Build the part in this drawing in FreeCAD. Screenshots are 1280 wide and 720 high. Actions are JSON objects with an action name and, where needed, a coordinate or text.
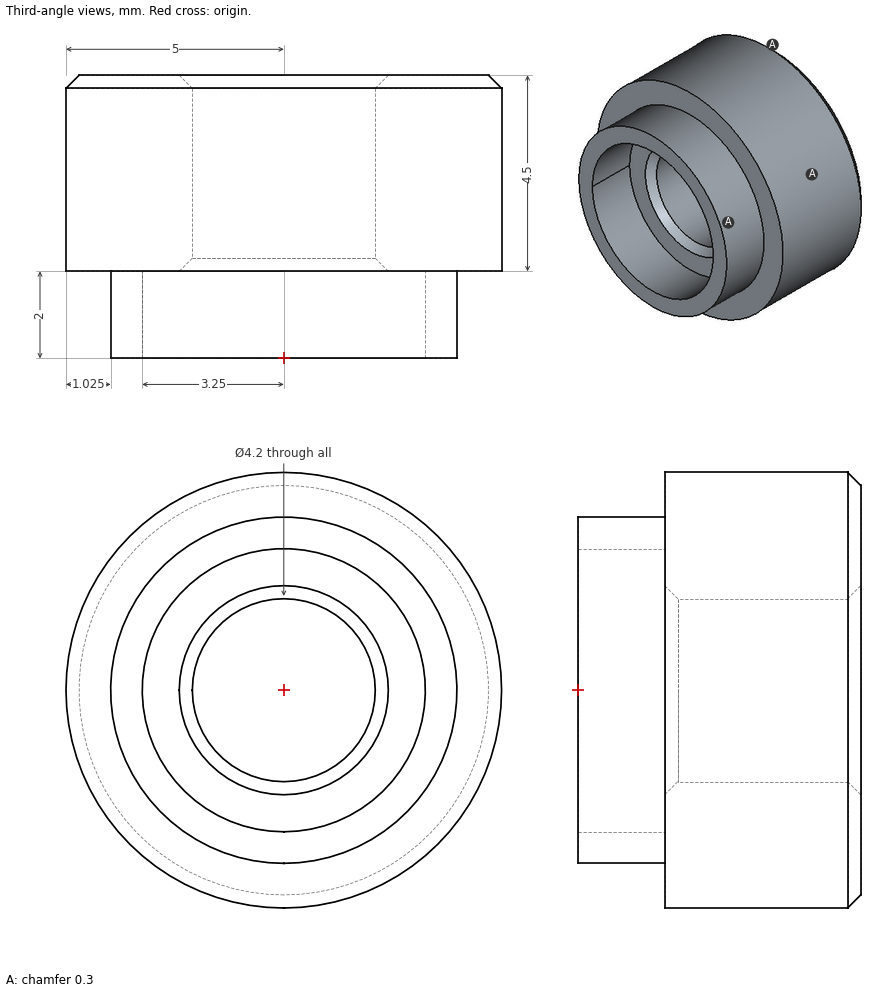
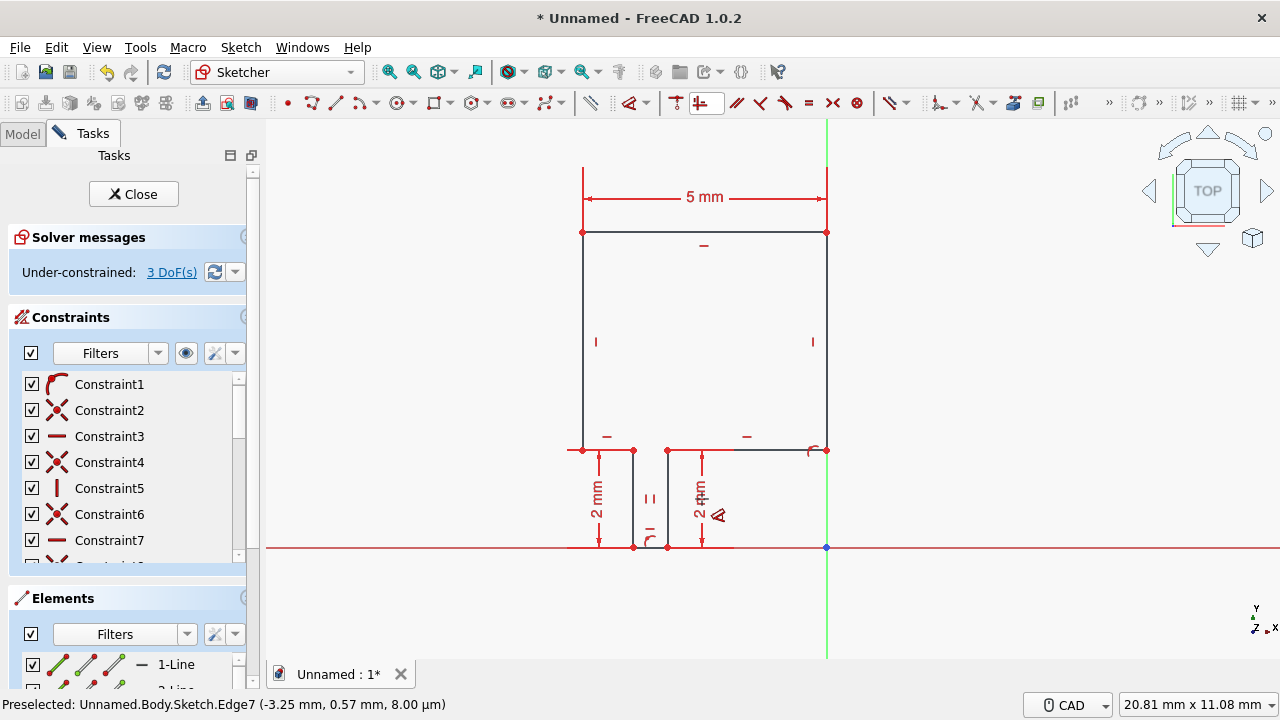
{"action": "left_click", "coordinate": [827, 385]}
{"action": "left_click", "coordinate": [861, 341]}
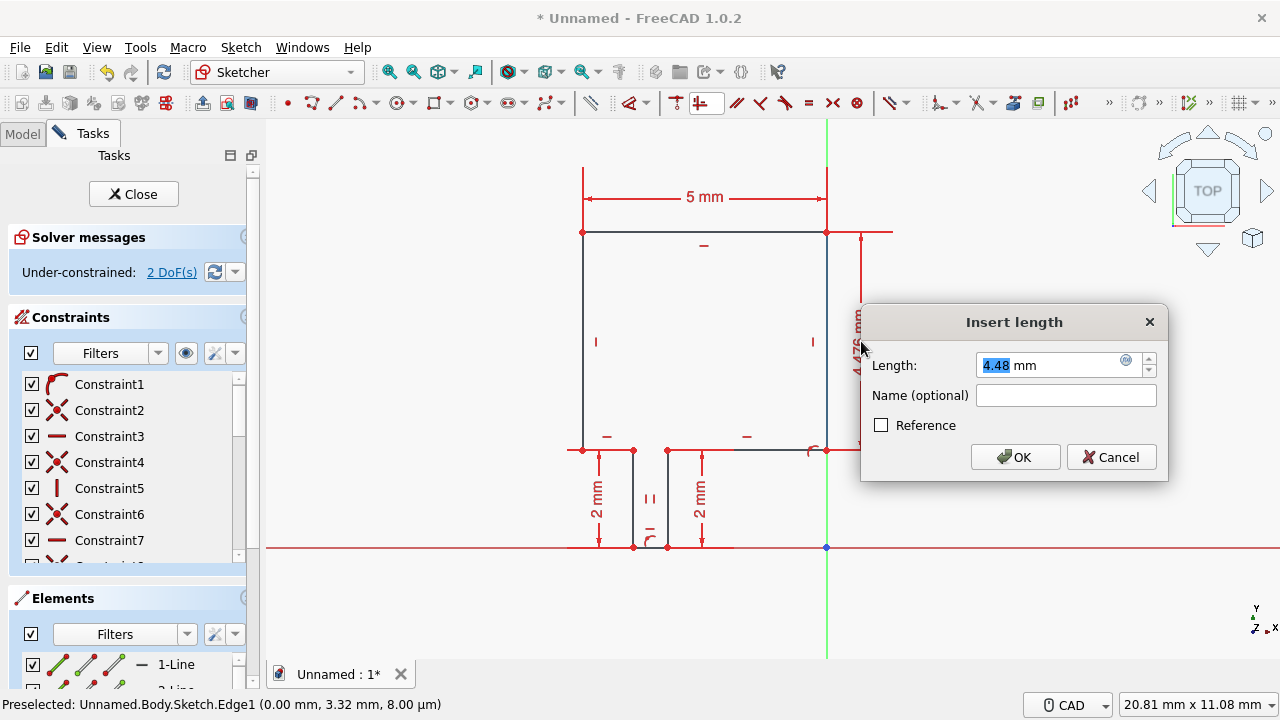
{"action": "type", "text": "4.5"}
{"action": "key", "text": "Return"}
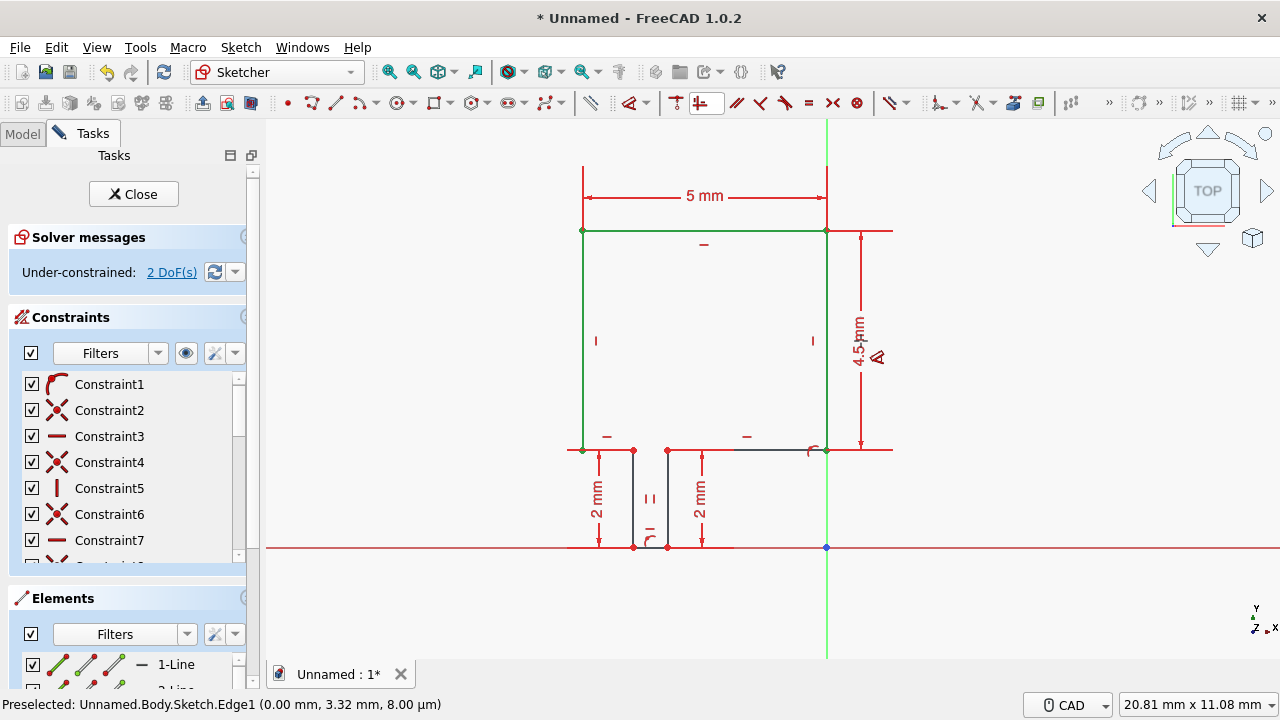
{"action": "left_click", "coordinate": [715, 450]}
{"action": "left_click", "coordinate": [784, 484]}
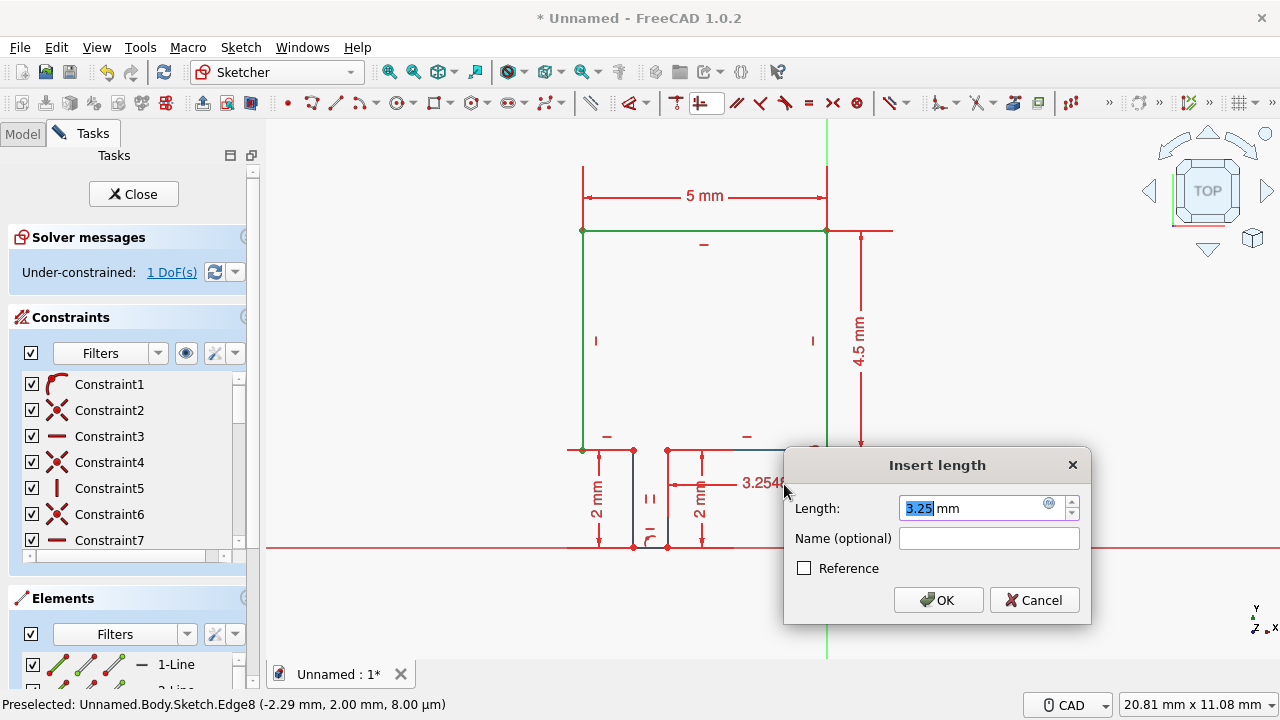
{"action": "type", "text": "3.25"}
{"action": "key", "text": "Return"}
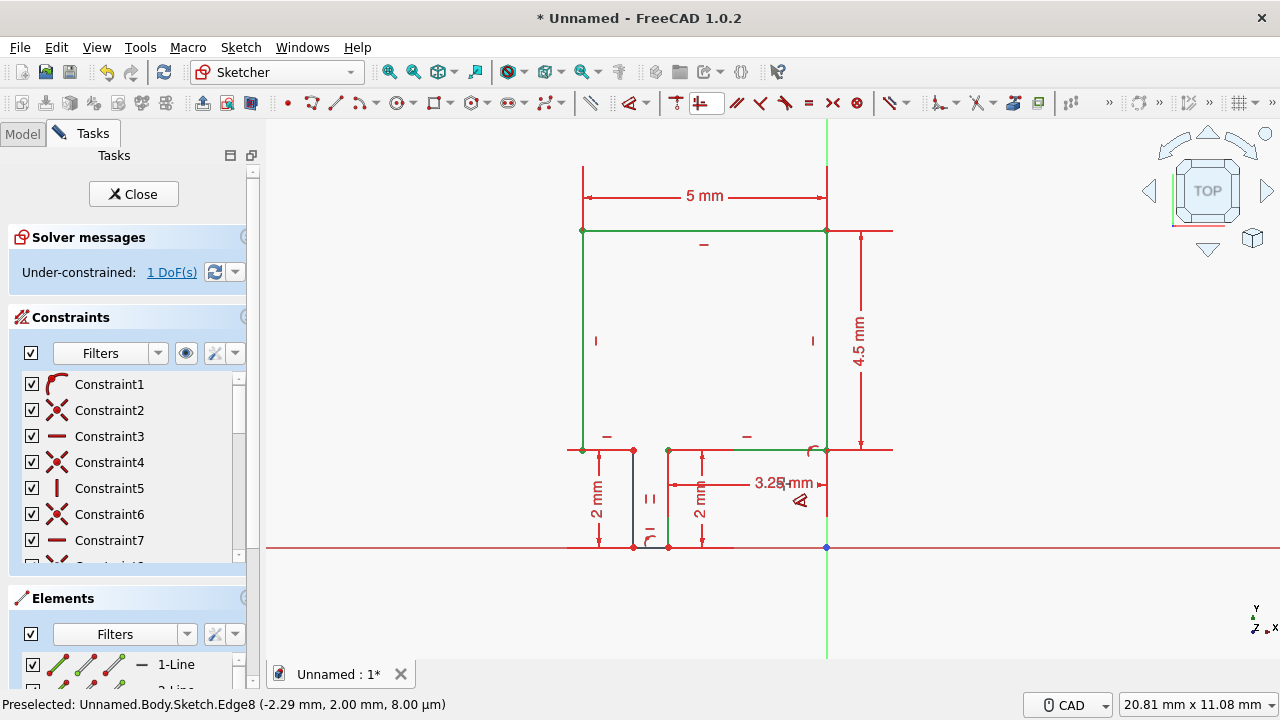
{"action": "left_click", "coordinate": [598, 450]}
{"action": "left_click", "coordinate": [608, 416]}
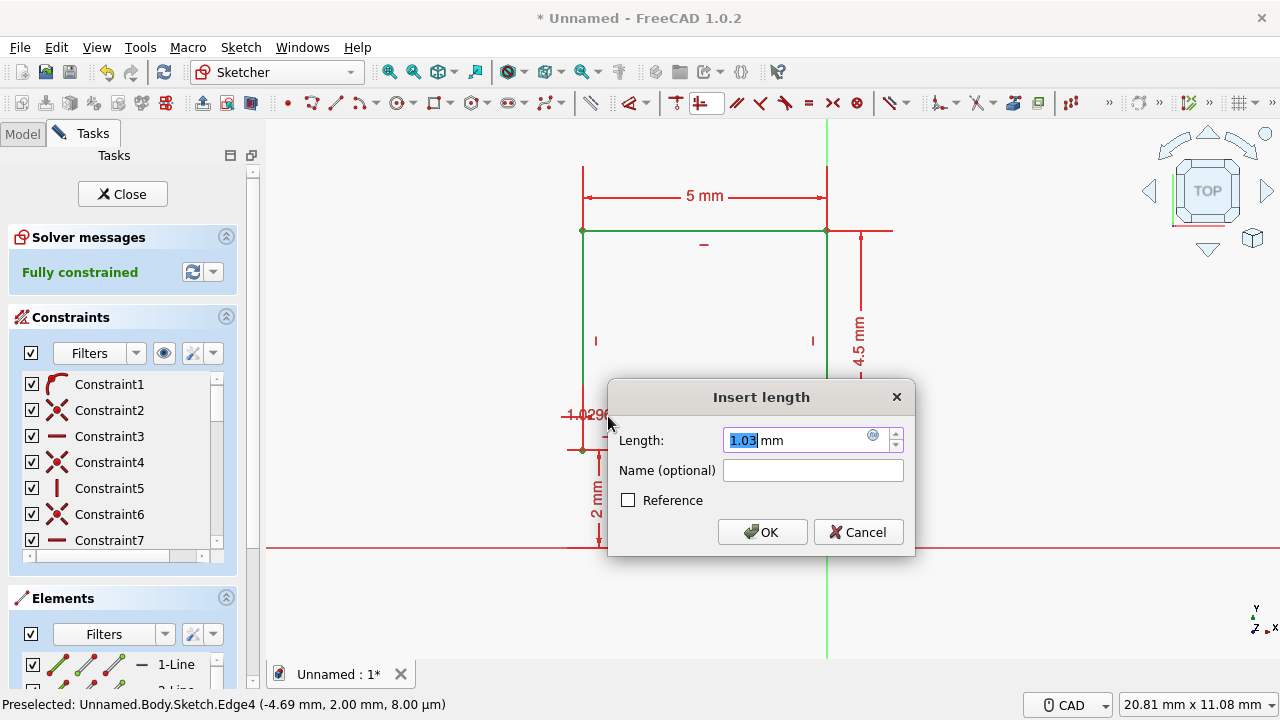
{"action": "type", "text": "1.025"}
{"action": "key", "text": "Return"}
{"action": "key", "text": "Escape"}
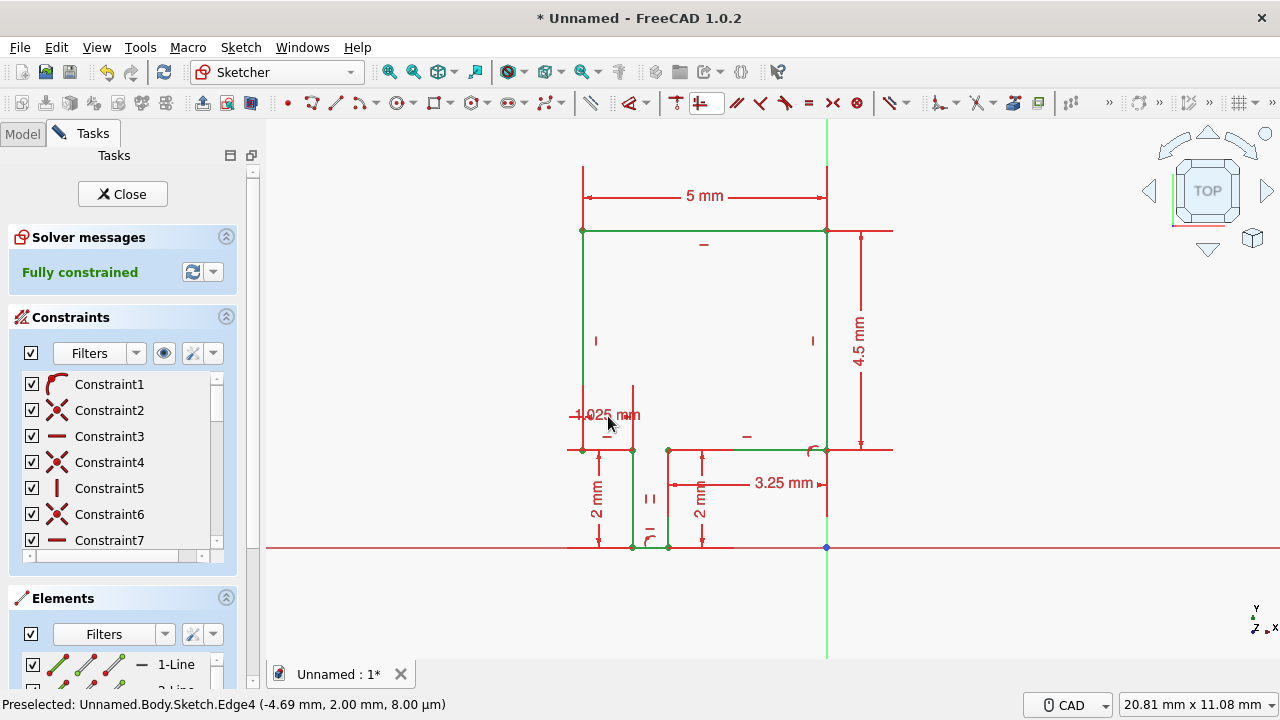
{"action": "left_click", "coordinate": [123, 194]}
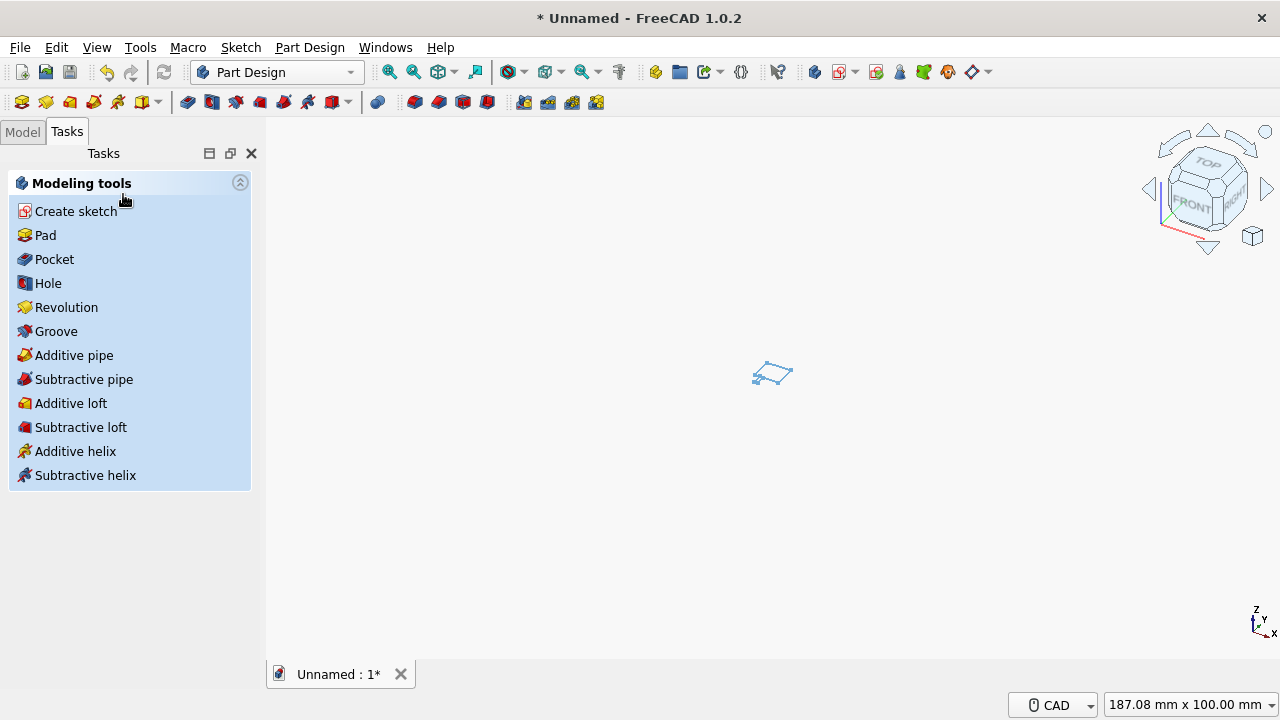
{"action": "left_click", "coordinate": [46, 102]}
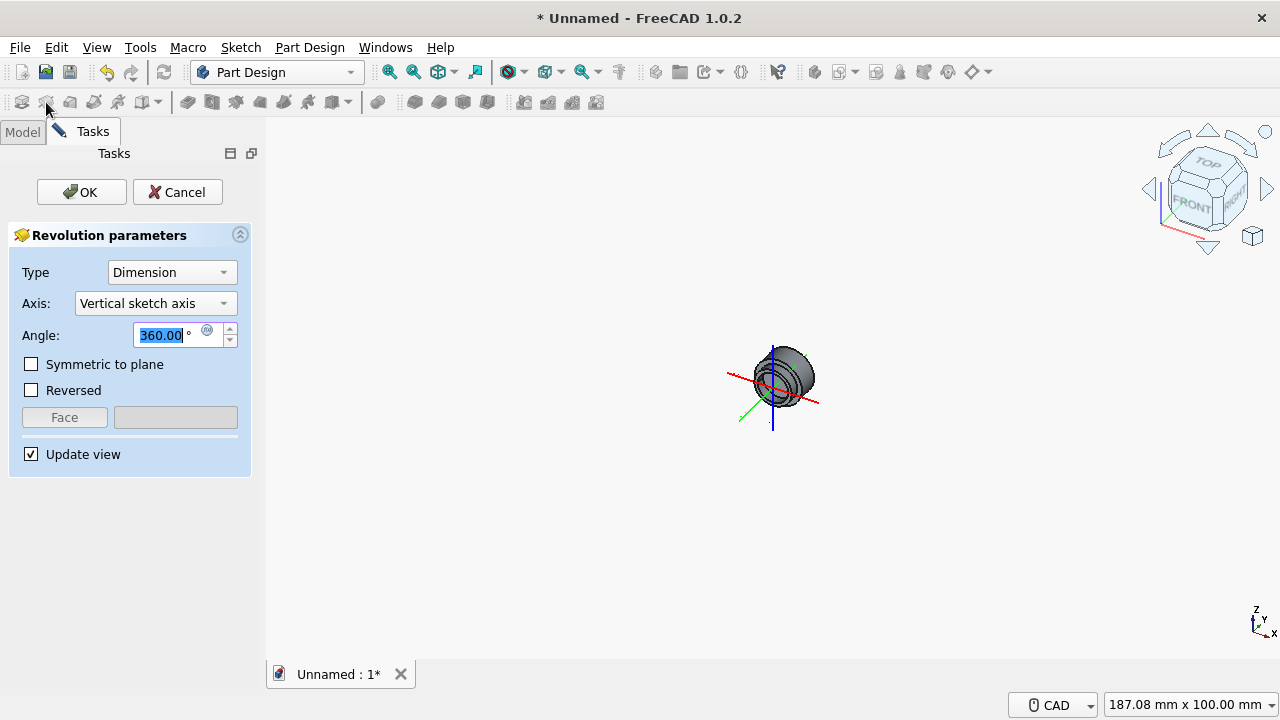
{"action": "left_click", "coordinate": [82, 192]}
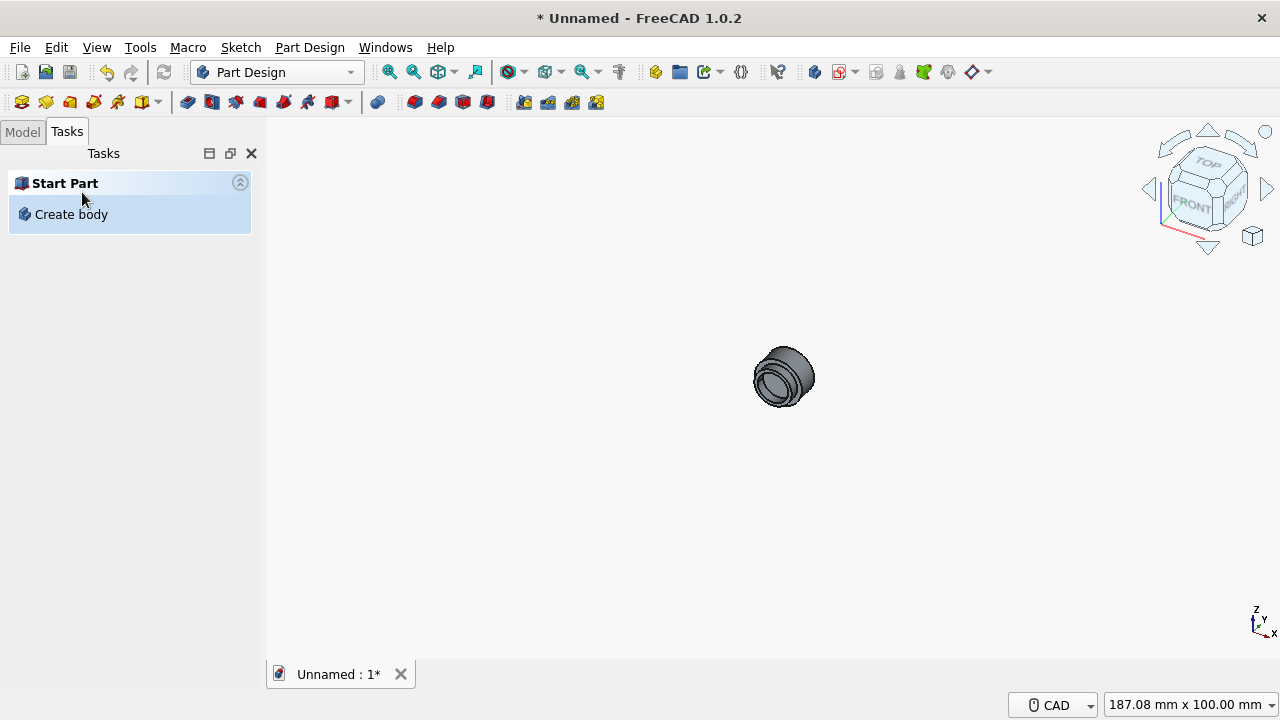
{"action": "left_click", "coordinate": [390, 72]}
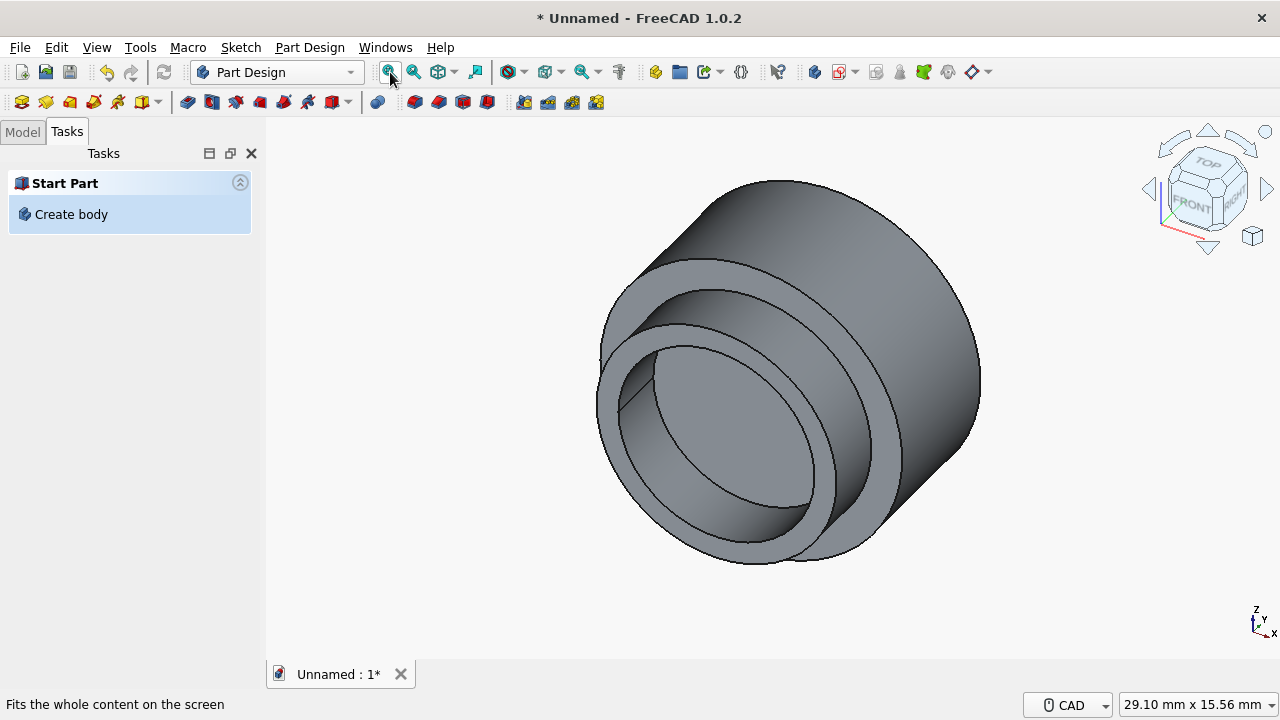
{"action": "key", "text": "4"}